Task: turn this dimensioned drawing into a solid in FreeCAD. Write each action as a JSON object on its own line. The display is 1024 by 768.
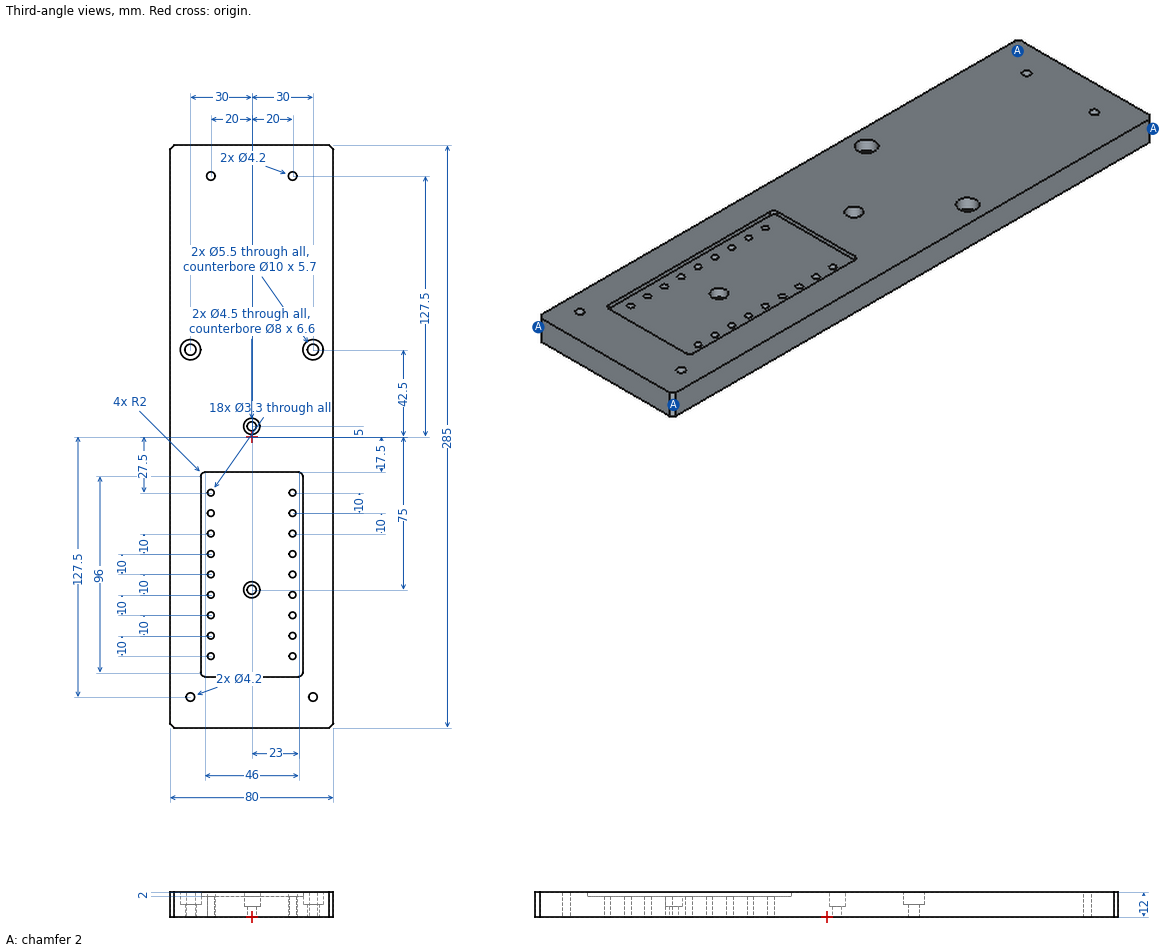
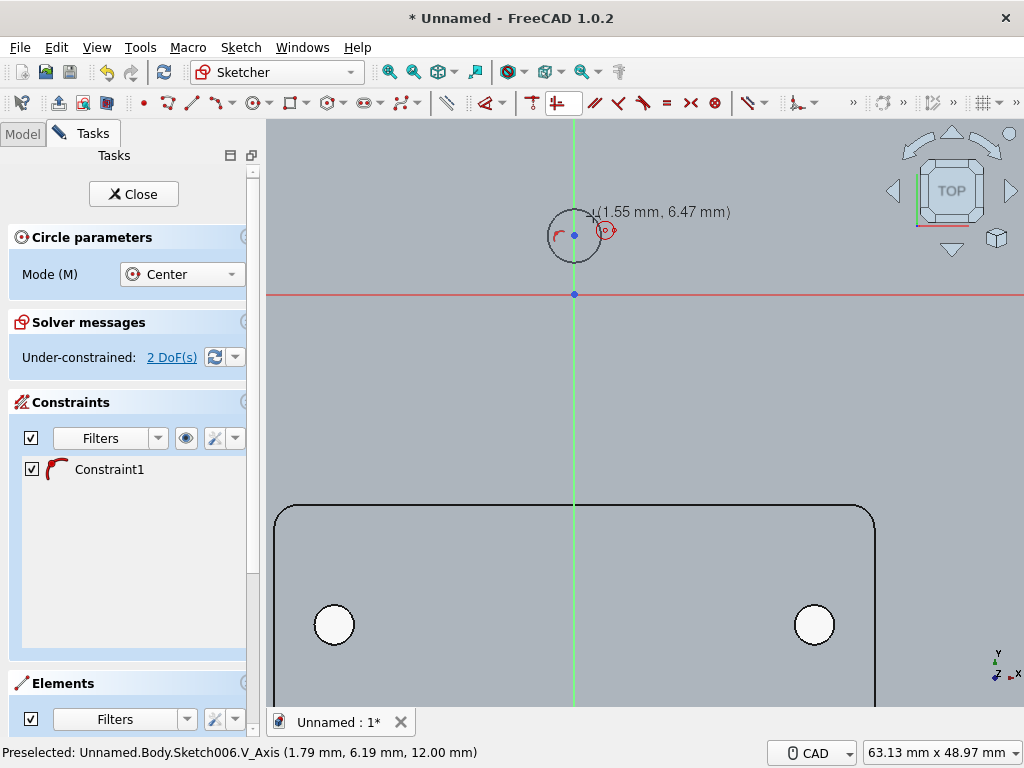
{"action": "scroll", "coordinate": [578, 237], "scroll_direction": "down", "scroll_amount": 5}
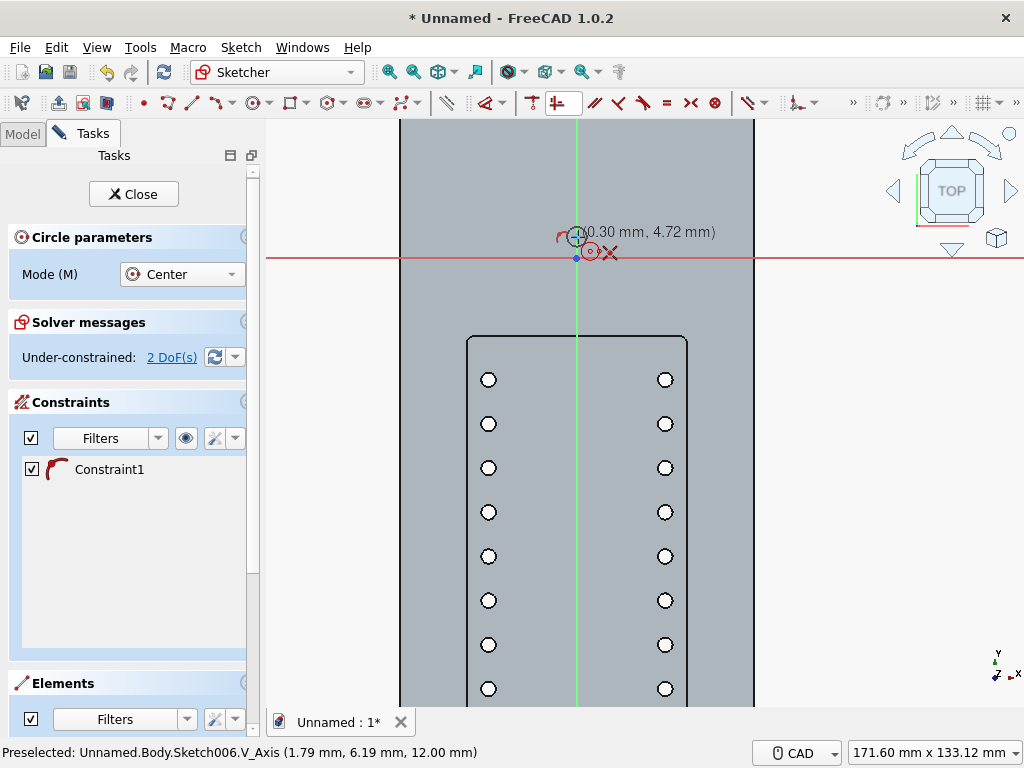
{"action": "scroll", "coordinate": [577, 590], "scroll_direction": "up", "scroll_amount": 5}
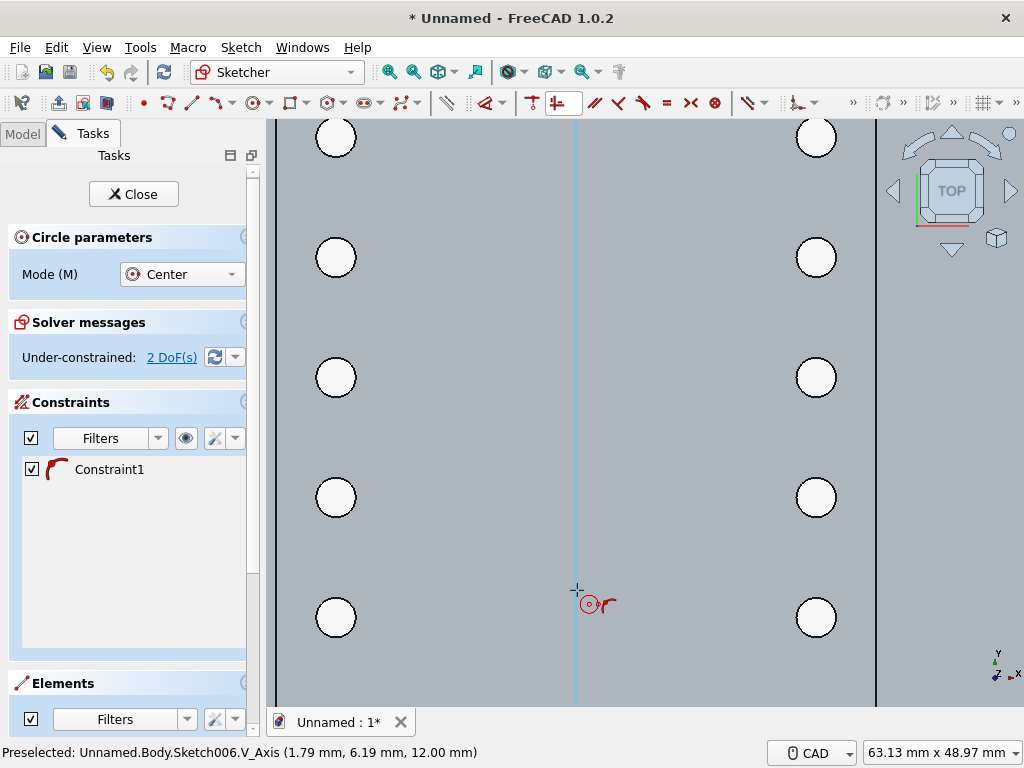
{"action": "left_click", "coordinate": [576, 588]}
{"action": "left_click", "coordinate": [595, 568]}
{"action": "key", "text": "Escape"}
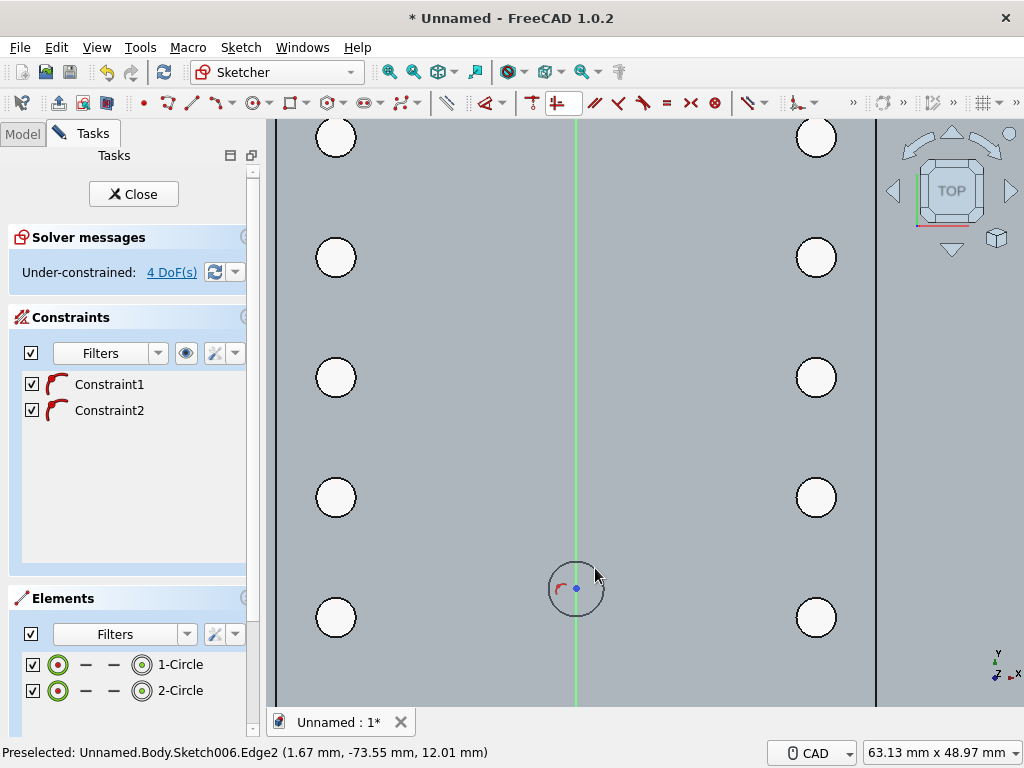
{"action": "scroll", "coordinate": [577, 591], "scroll_direction": "down", "scroll_amount": 5}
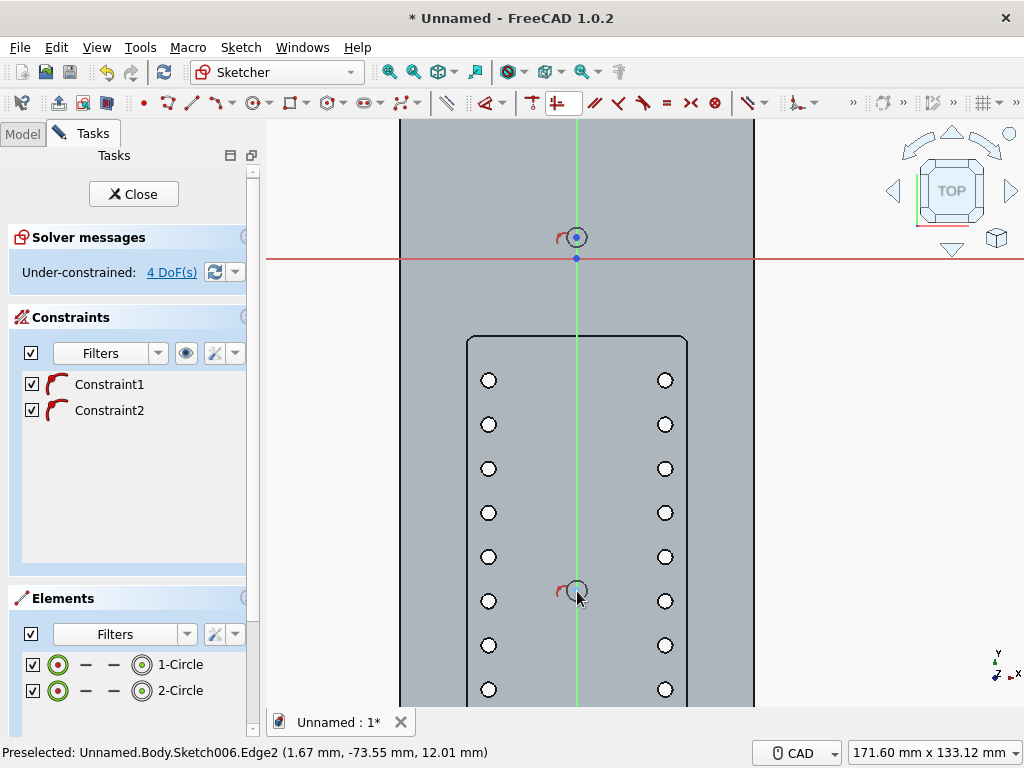
{"action": "scroll", "coordinate": [584, 230], "scroll_direction": "up", "scroll_amount": 4}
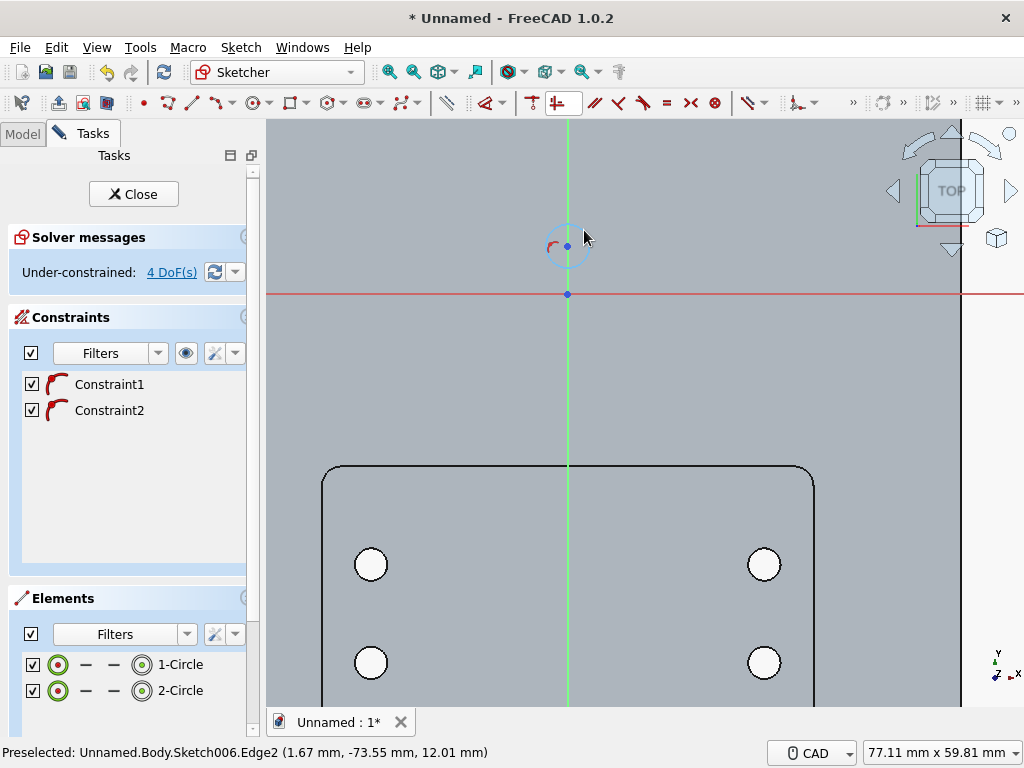
{"action": "left_click", "coordinate": [583, 231]}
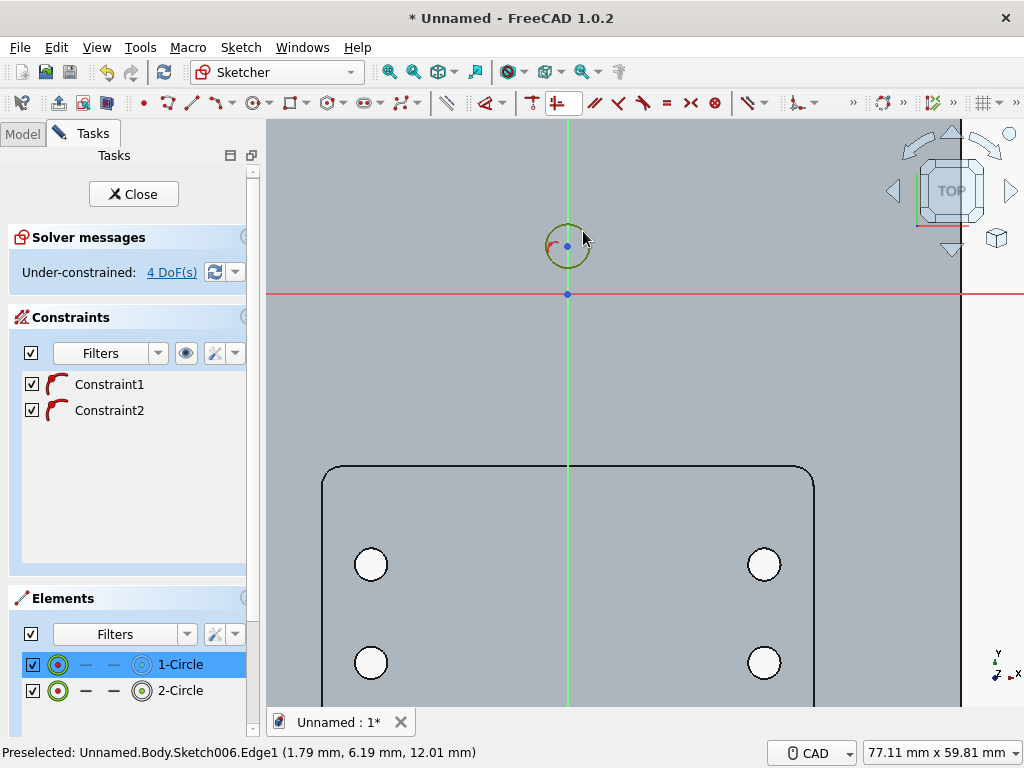
{"action": "scroll", "coordinate": [584, 229], "scroll_direction": "down", "scroll_amount": 4}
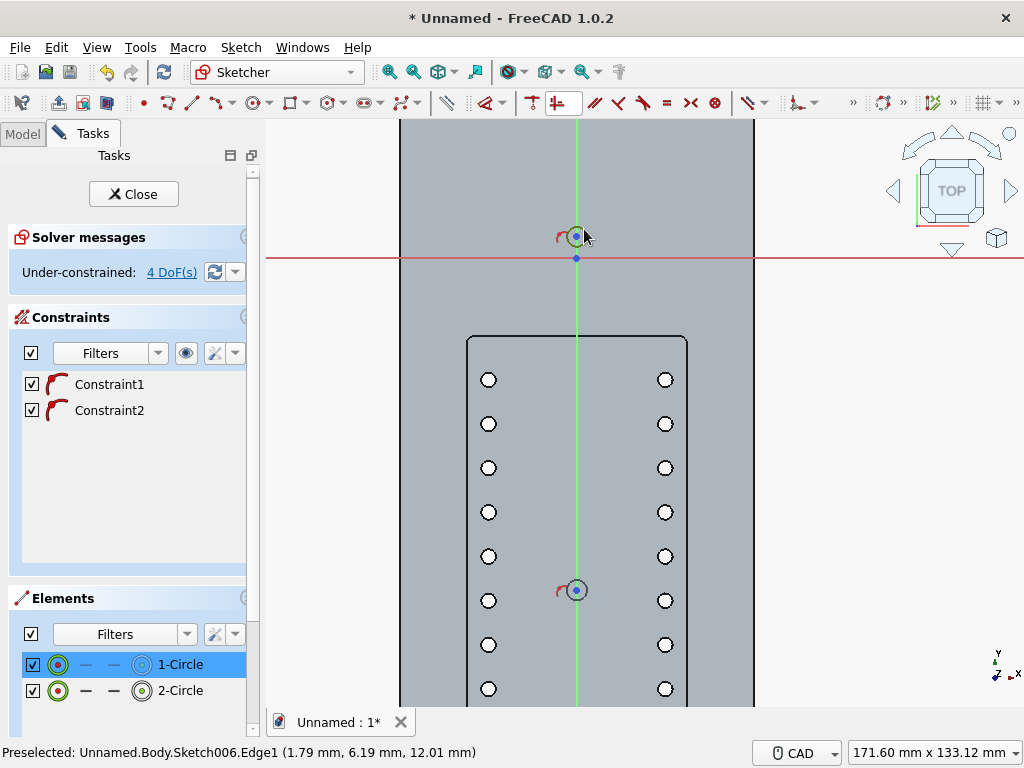
{"action": "scroll", "coordinate": [584, 583], "scroll_direction": "up", "scroll_amount": 4}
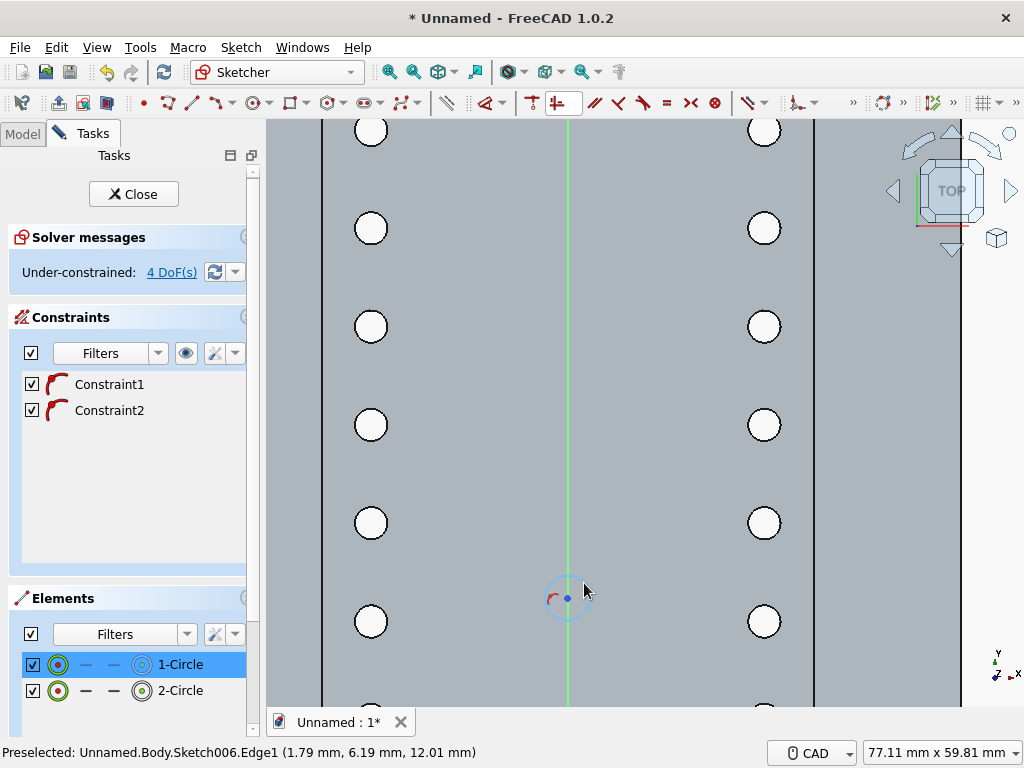
{"action": "left_click", "coordinate": [584, 582]}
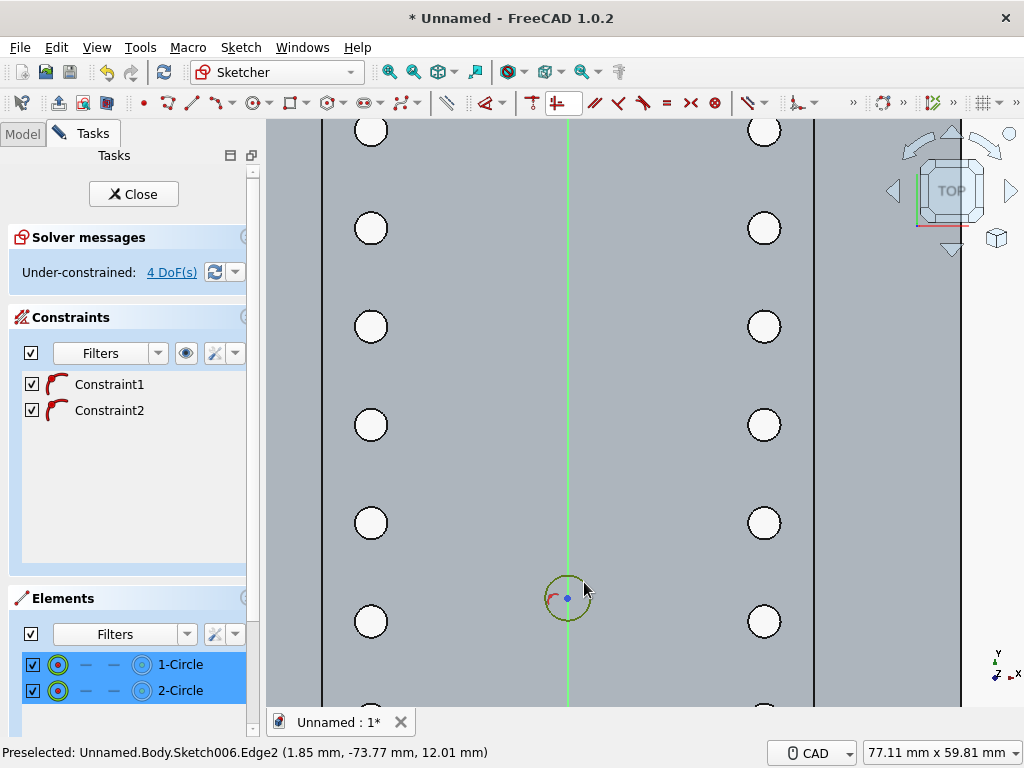
{"action": "left_click", "coordinate": [668, 104]}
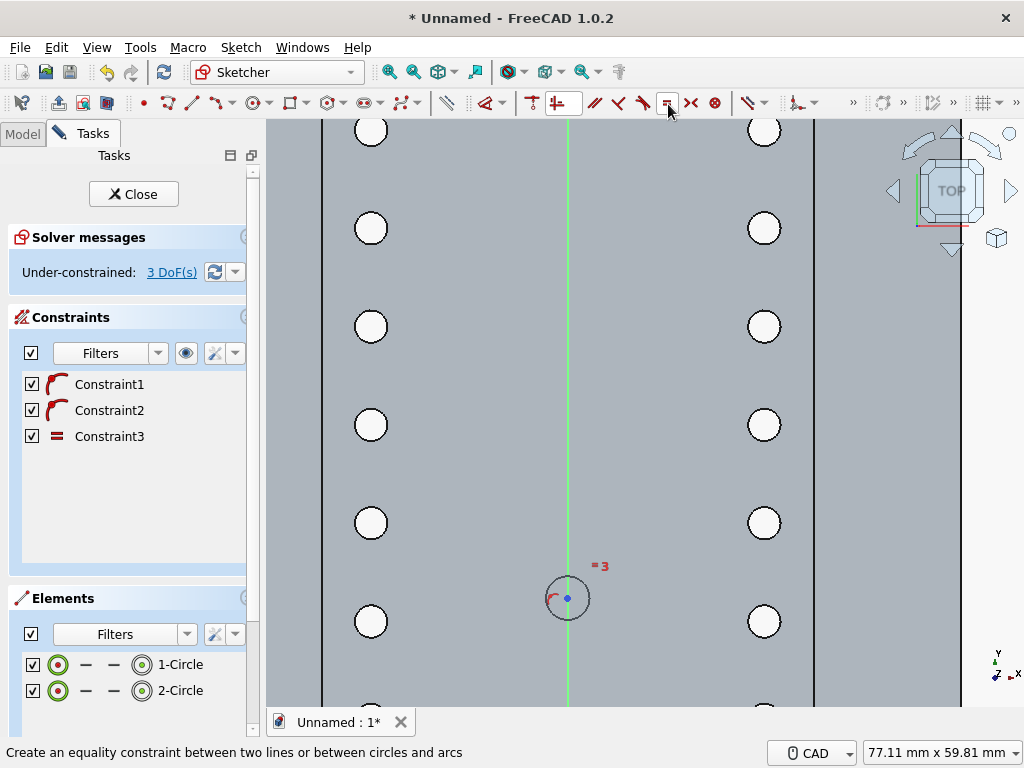
{"action": "left_click", "coordinate": [486, 104]}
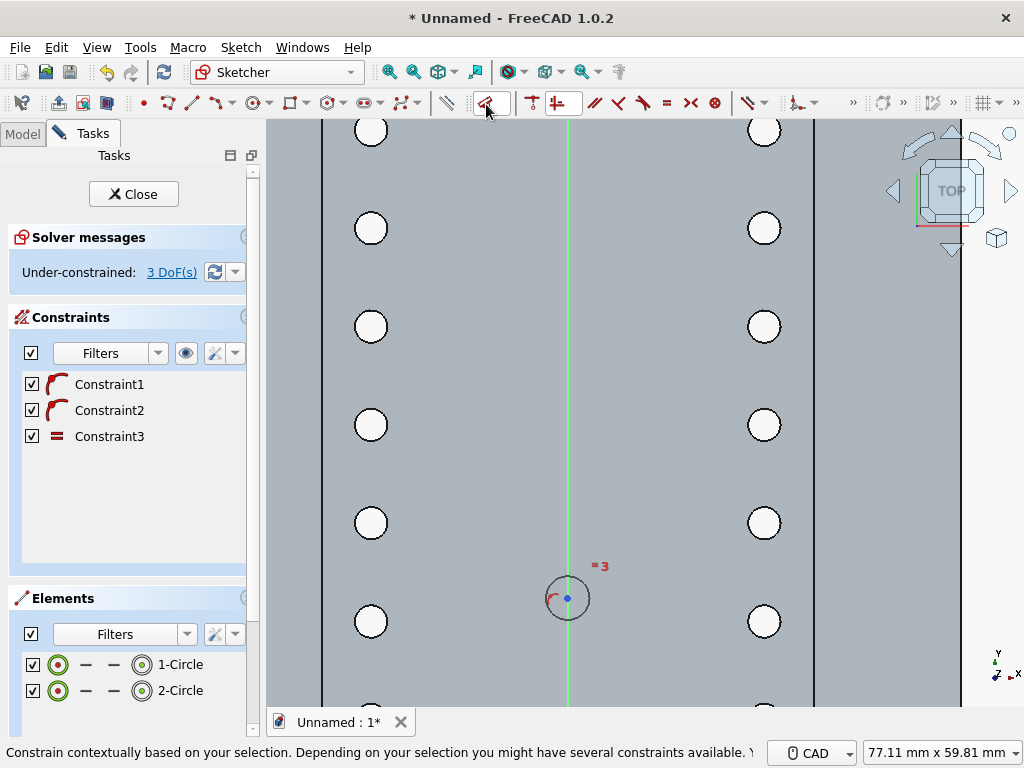
{"action": "scroll", "coordinate": [584, 584], "scroll_direction": "down", "scroll_amount": 4}